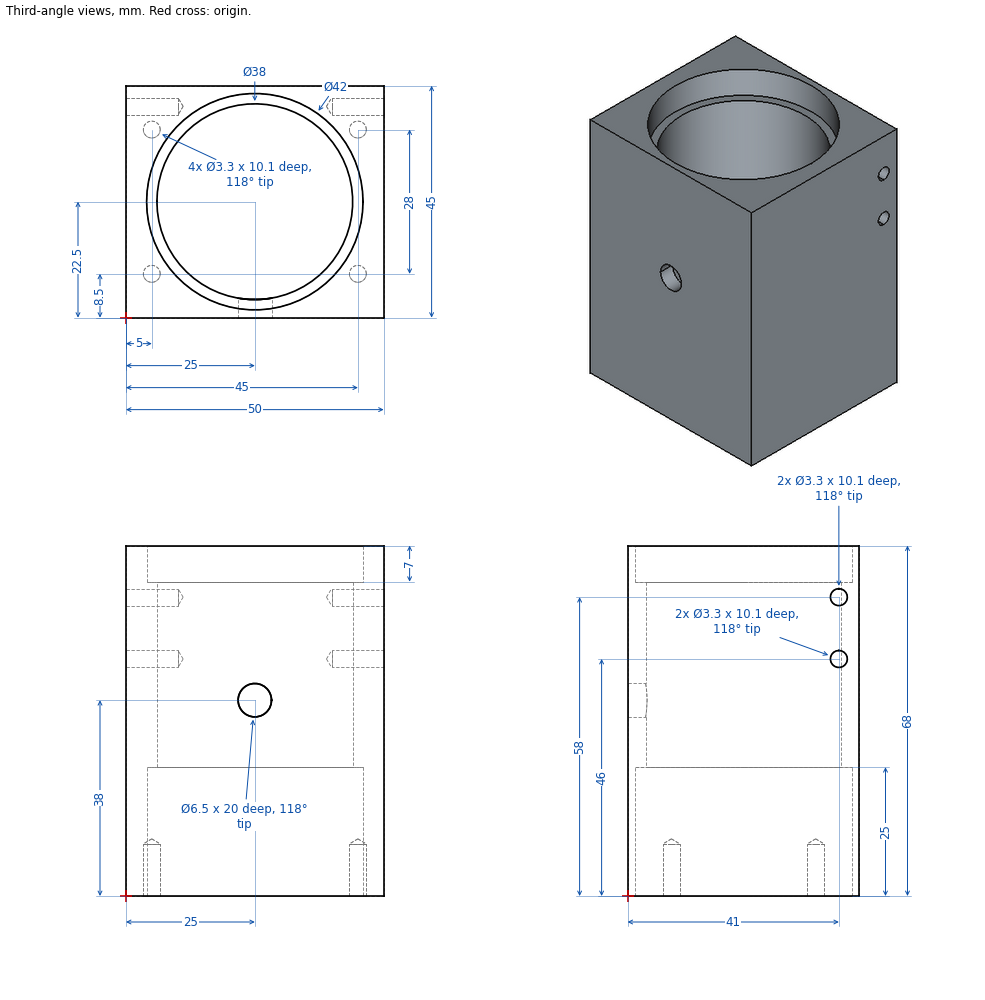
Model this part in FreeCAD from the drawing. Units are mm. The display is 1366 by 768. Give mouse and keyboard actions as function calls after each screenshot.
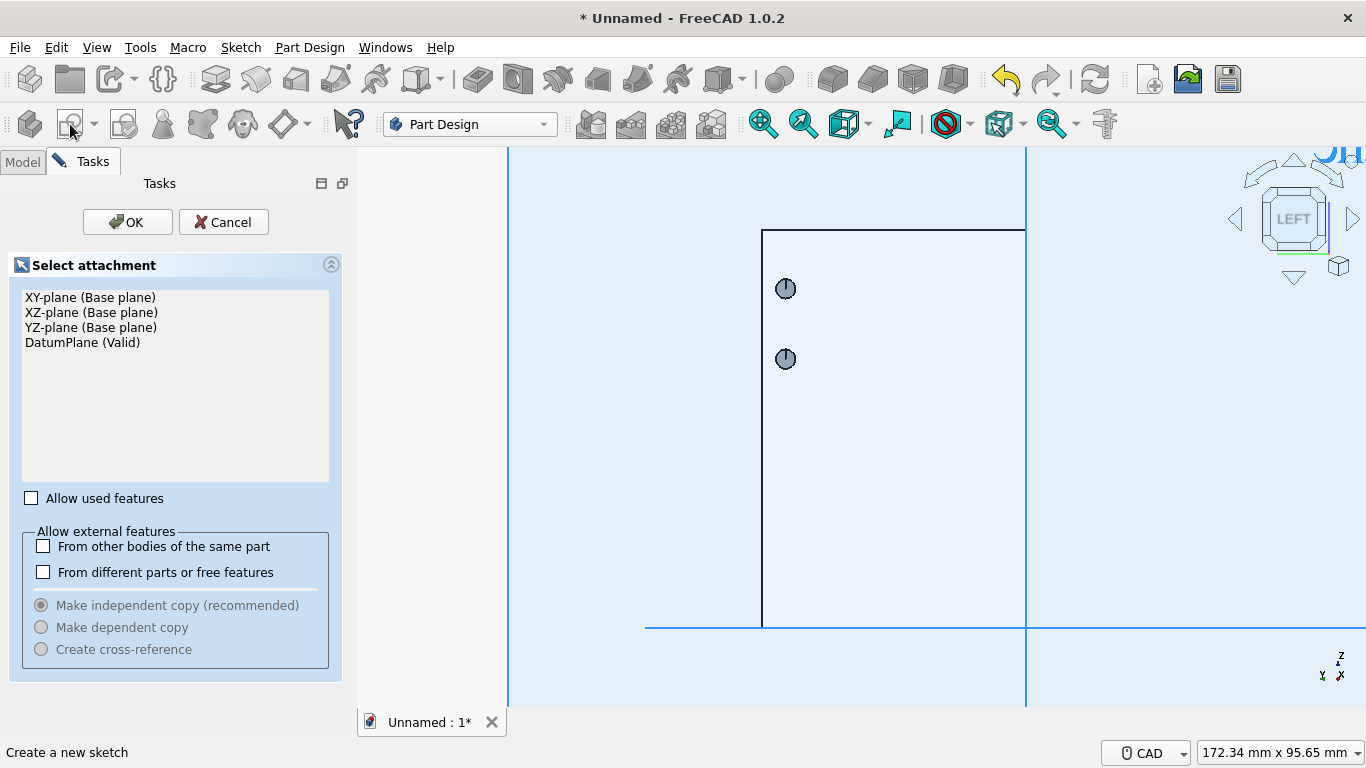
click(82, 312)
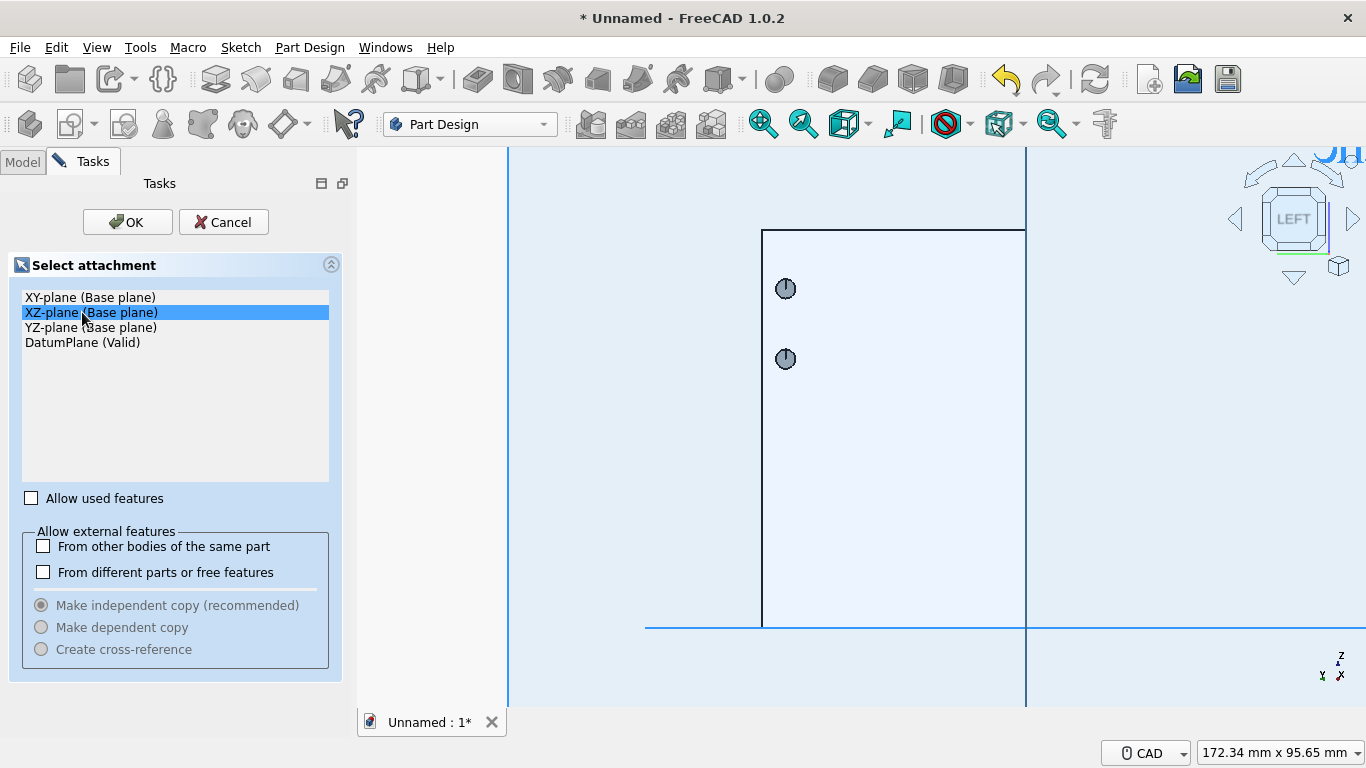
click(128, 222)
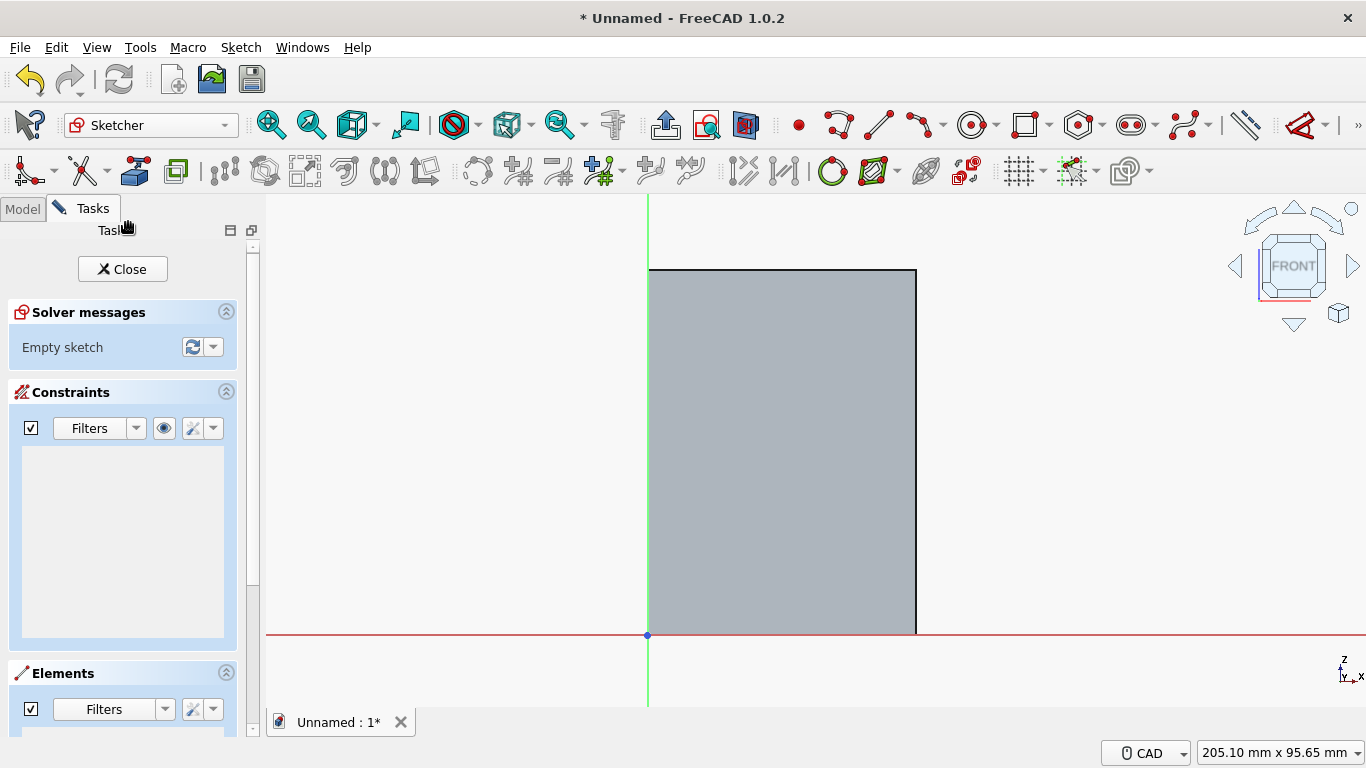
scroll(786, 429, up, 11)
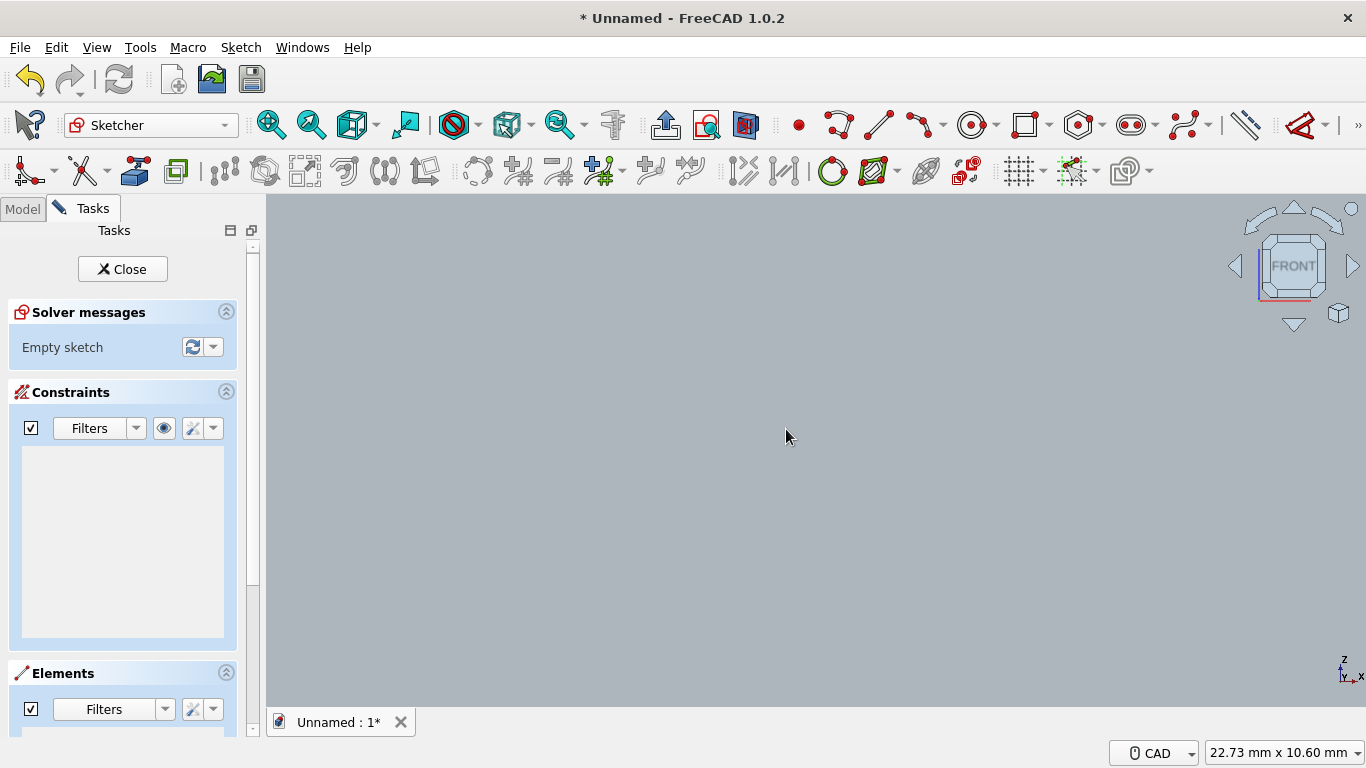
click(972, 126)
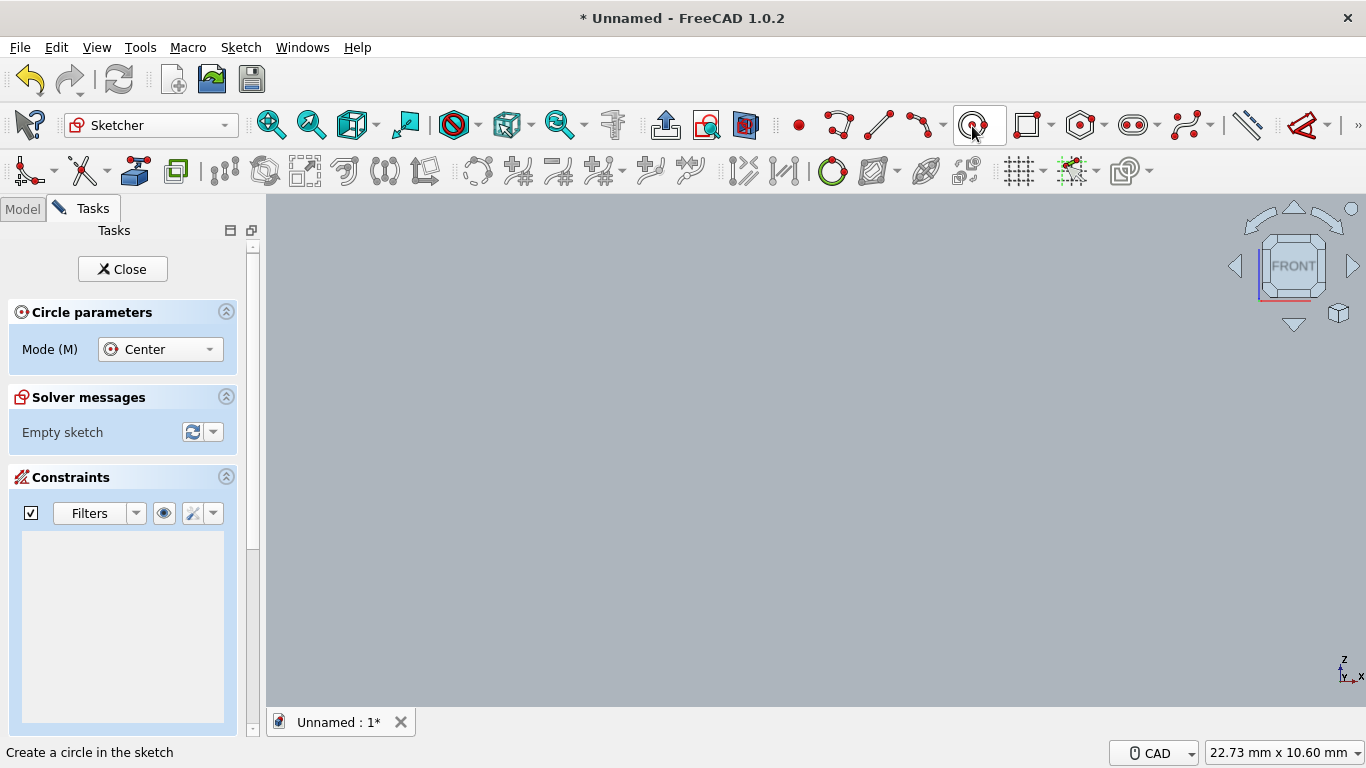
click(745, 446)
move(856, 334)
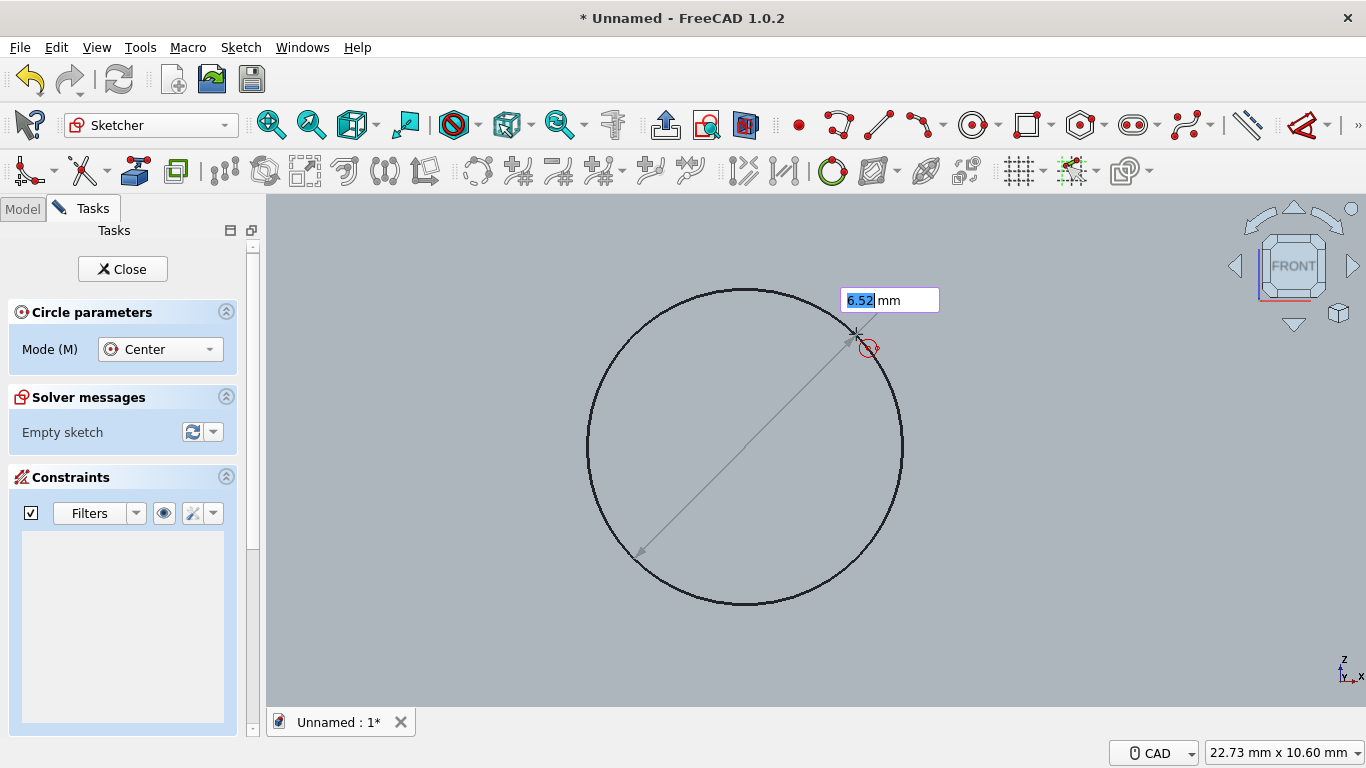
text(6.5)
key(Return)
key(Escape)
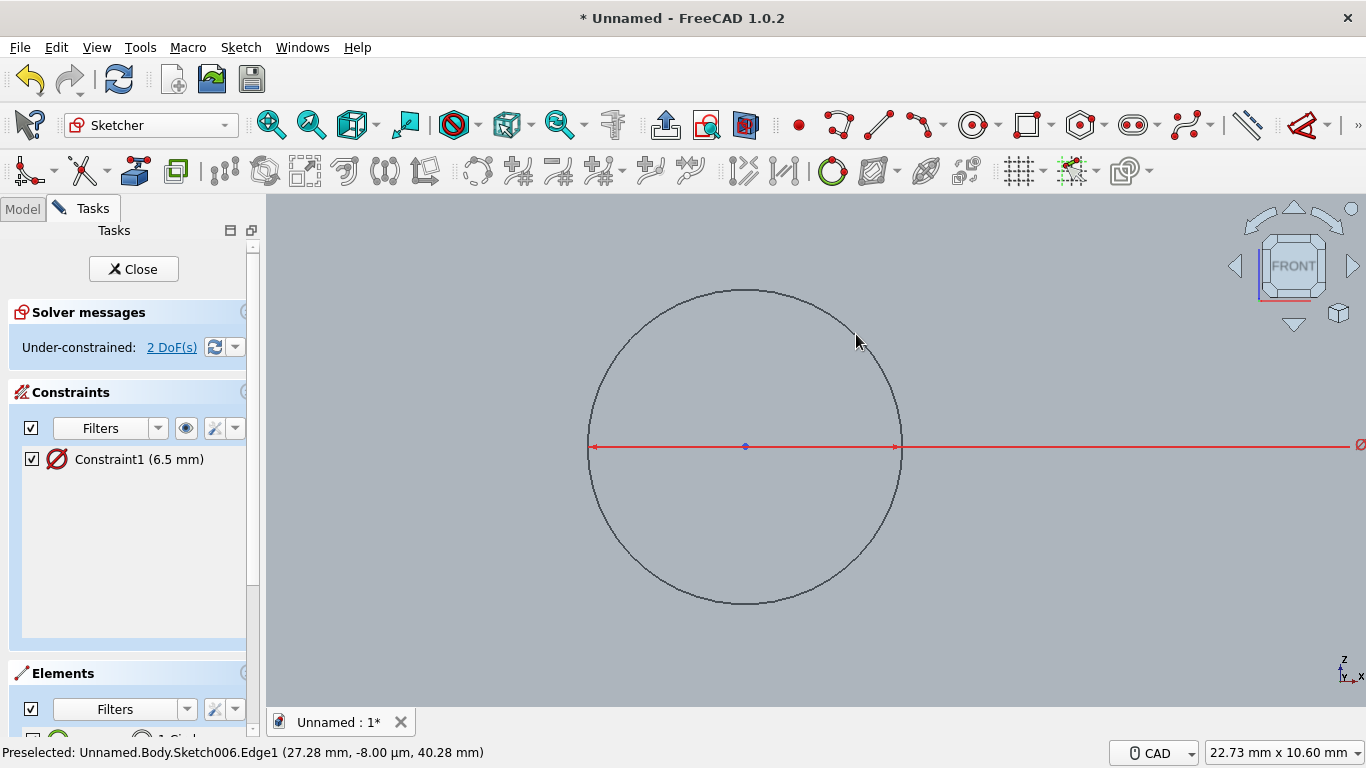
key(d)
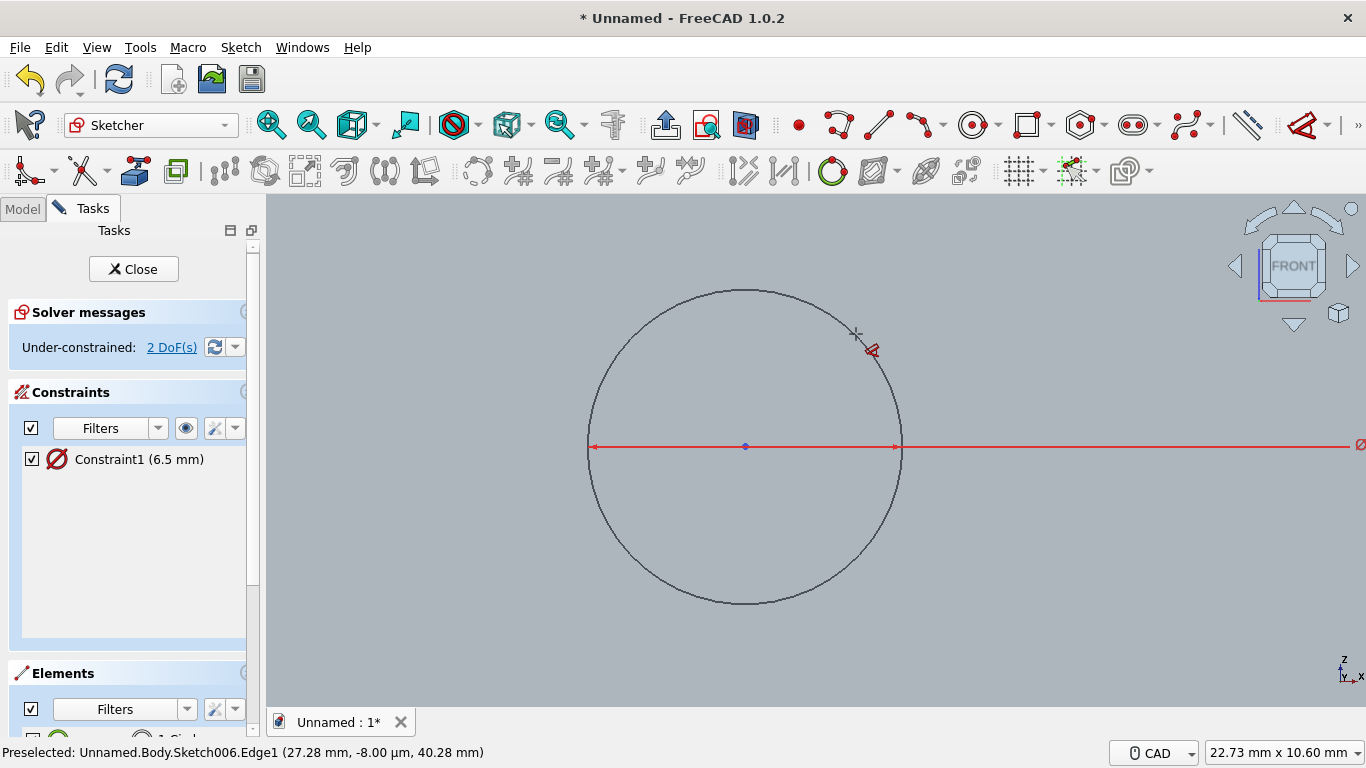
click(745, 447)
click(519, 413)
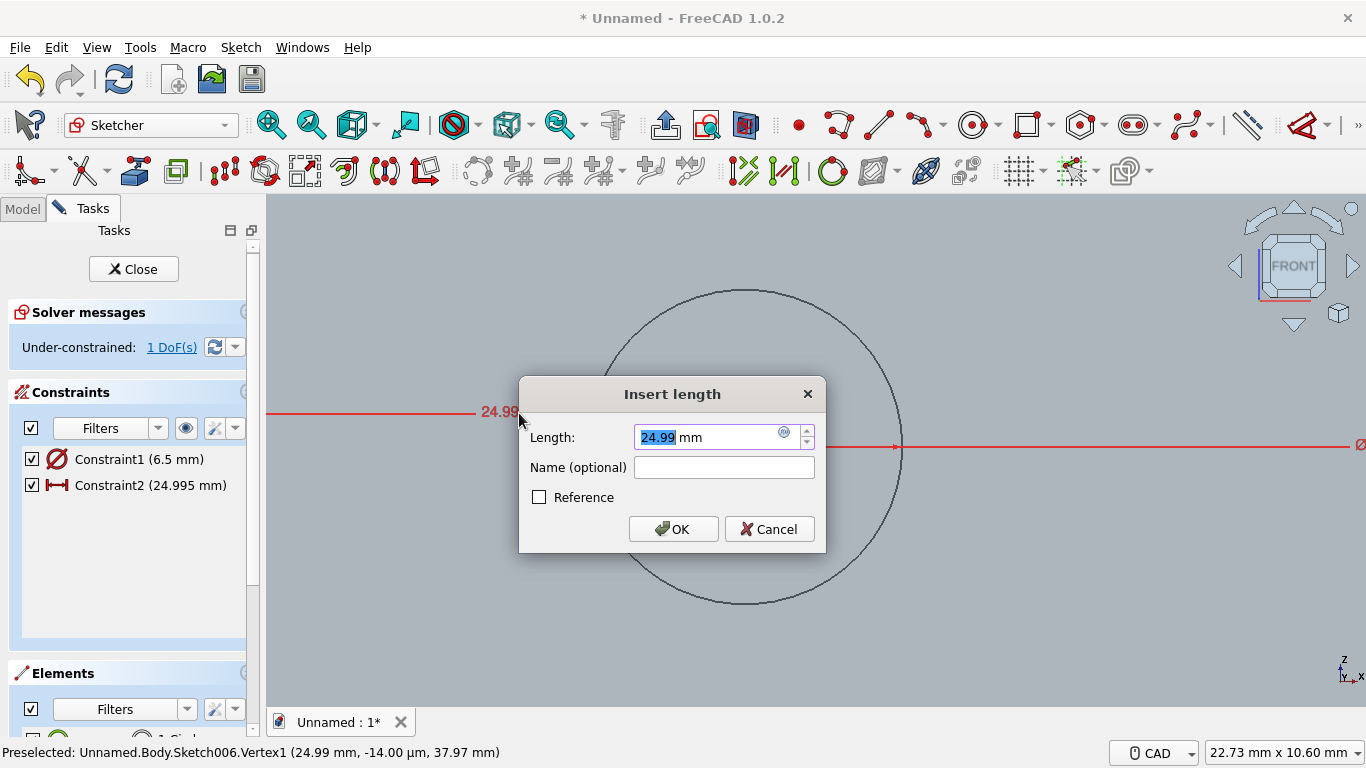
text(25)
key(Return)